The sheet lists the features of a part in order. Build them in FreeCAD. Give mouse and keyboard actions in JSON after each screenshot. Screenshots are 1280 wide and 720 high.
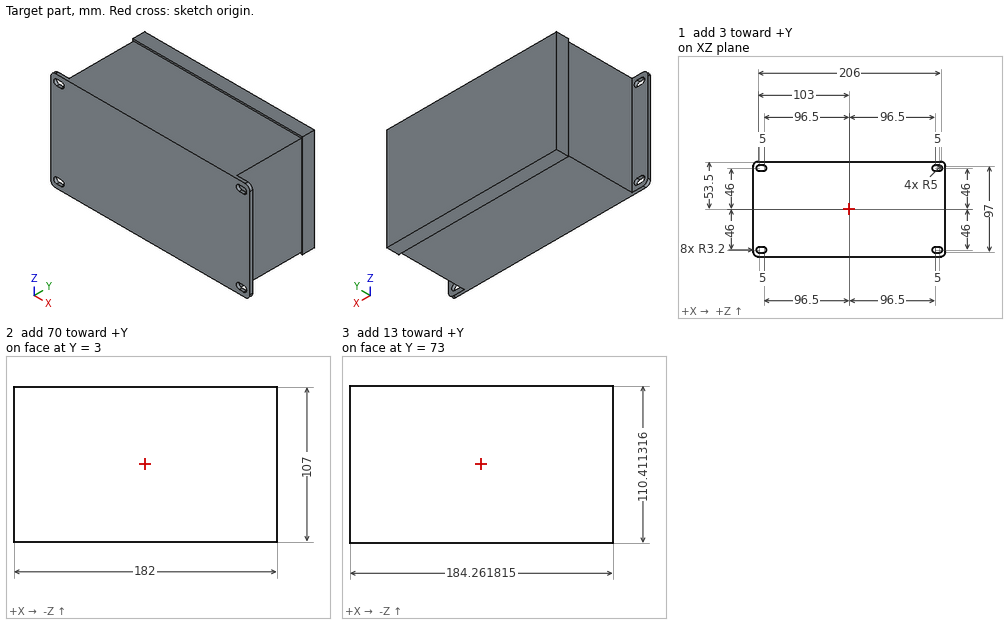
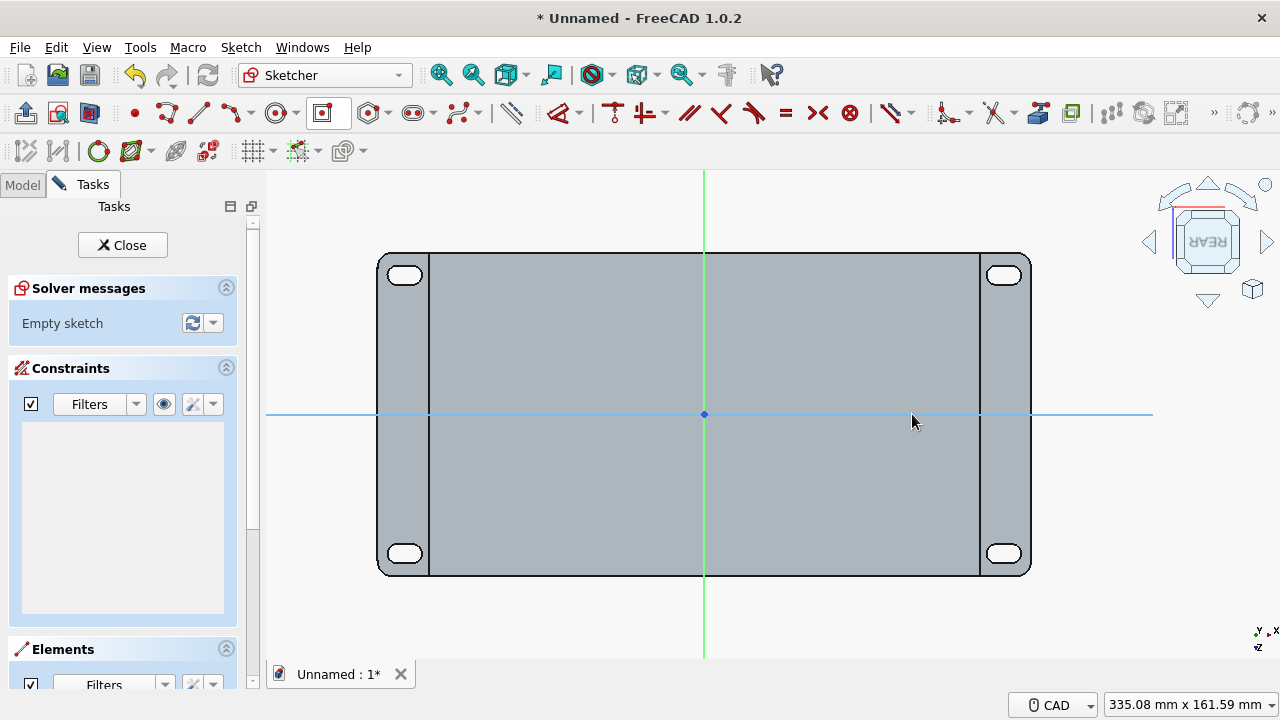
{"action": "left_click", "coordinate": [322, 114]}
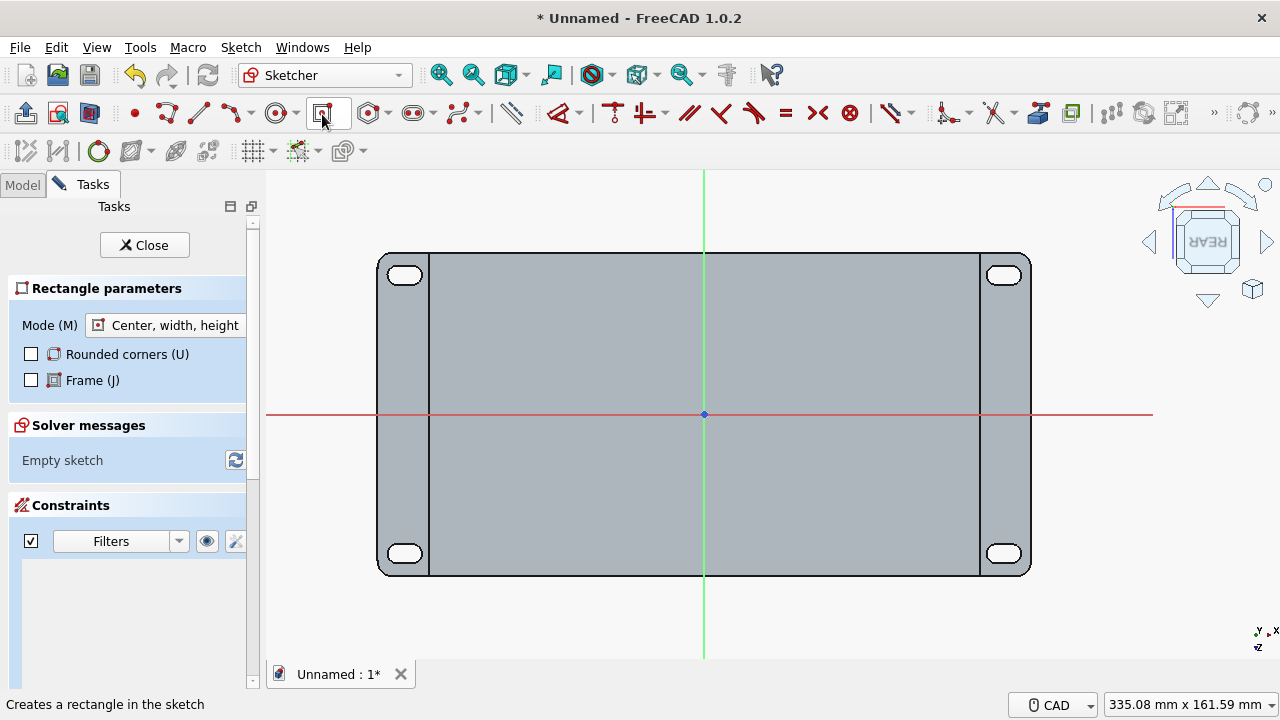
{"action": "left_click", "coordinate": [704, 414]}
{"action": "left_click", "coordinate": [983, 247]}
{"action": "key", "text": "Escape"}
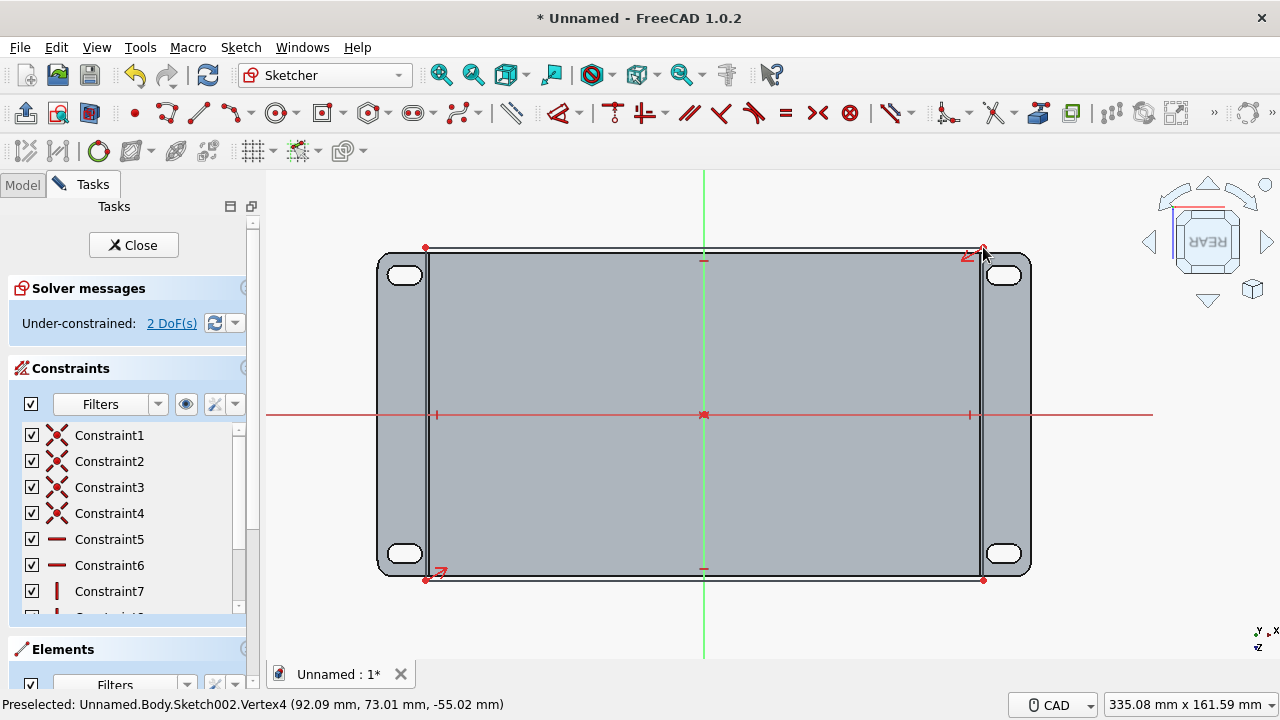
{"action": "left_click", "coordinate": [558, 114]}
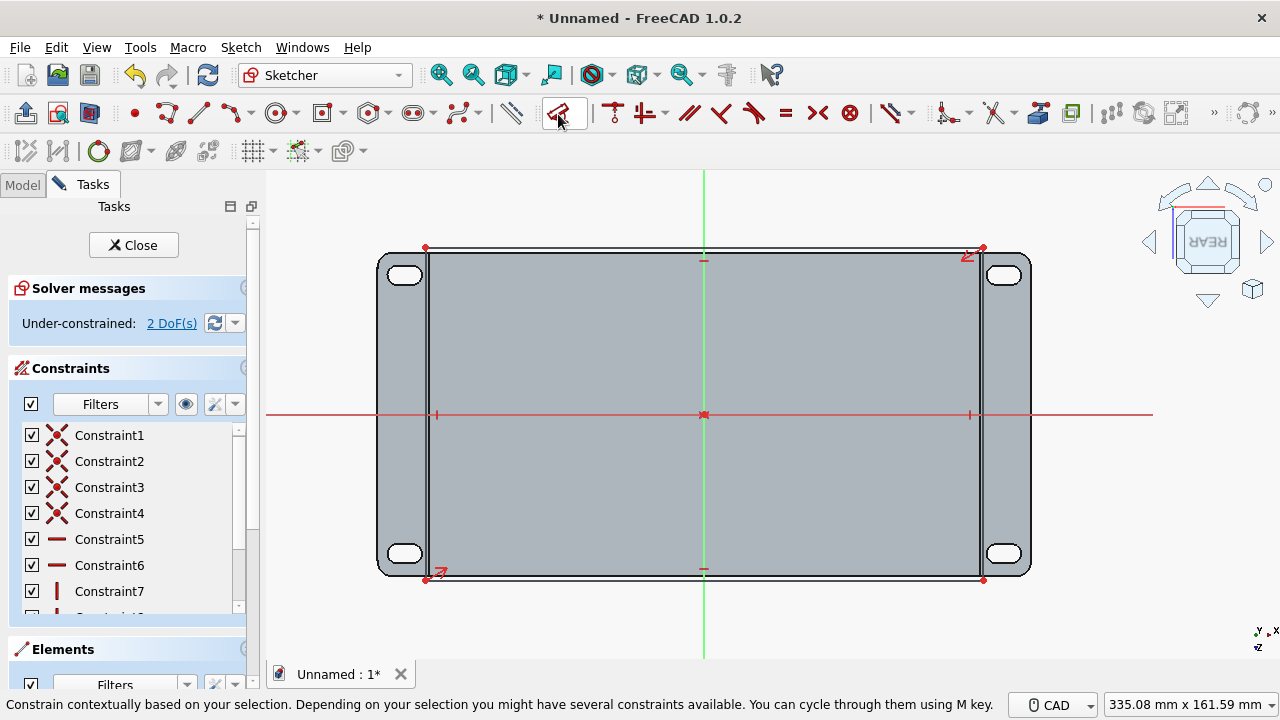
{"action": "left_click", "coordinate": [593, 581]}
{"action": "left_click", "coordinate": [576, 615]}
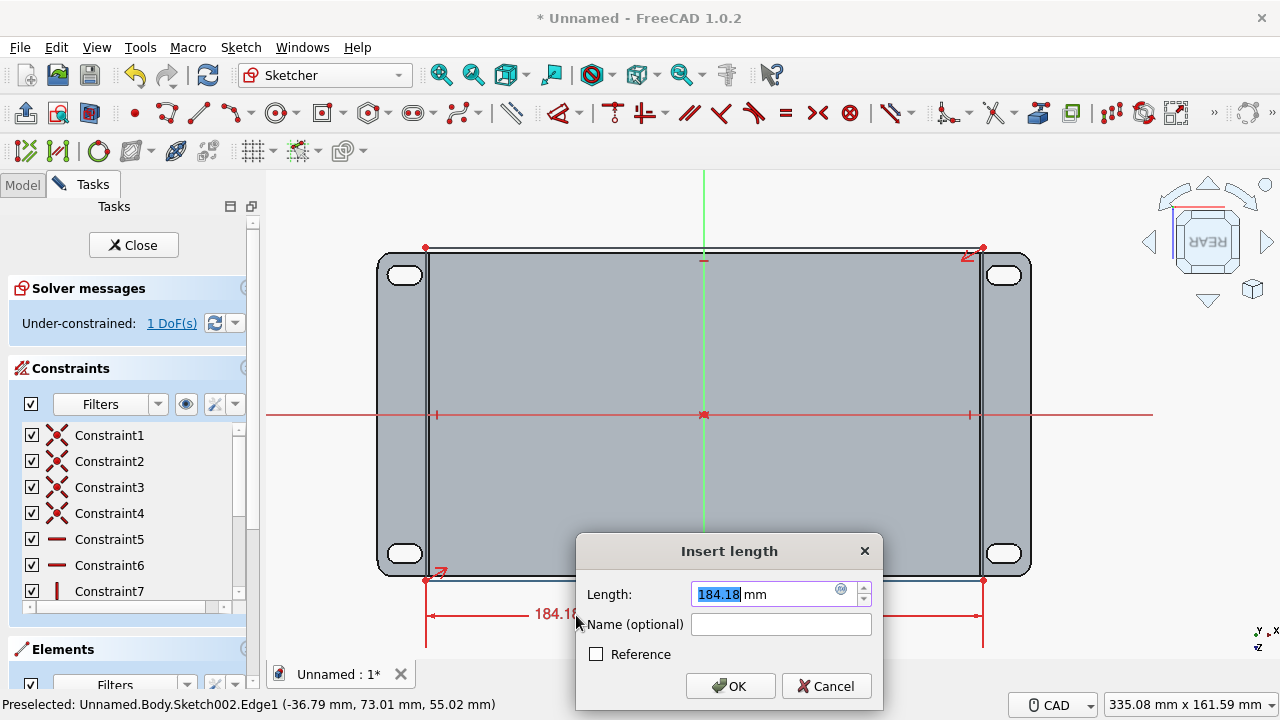
{"action": "type", "text": "184.261815"}
{"action": "key", "text": "Return"}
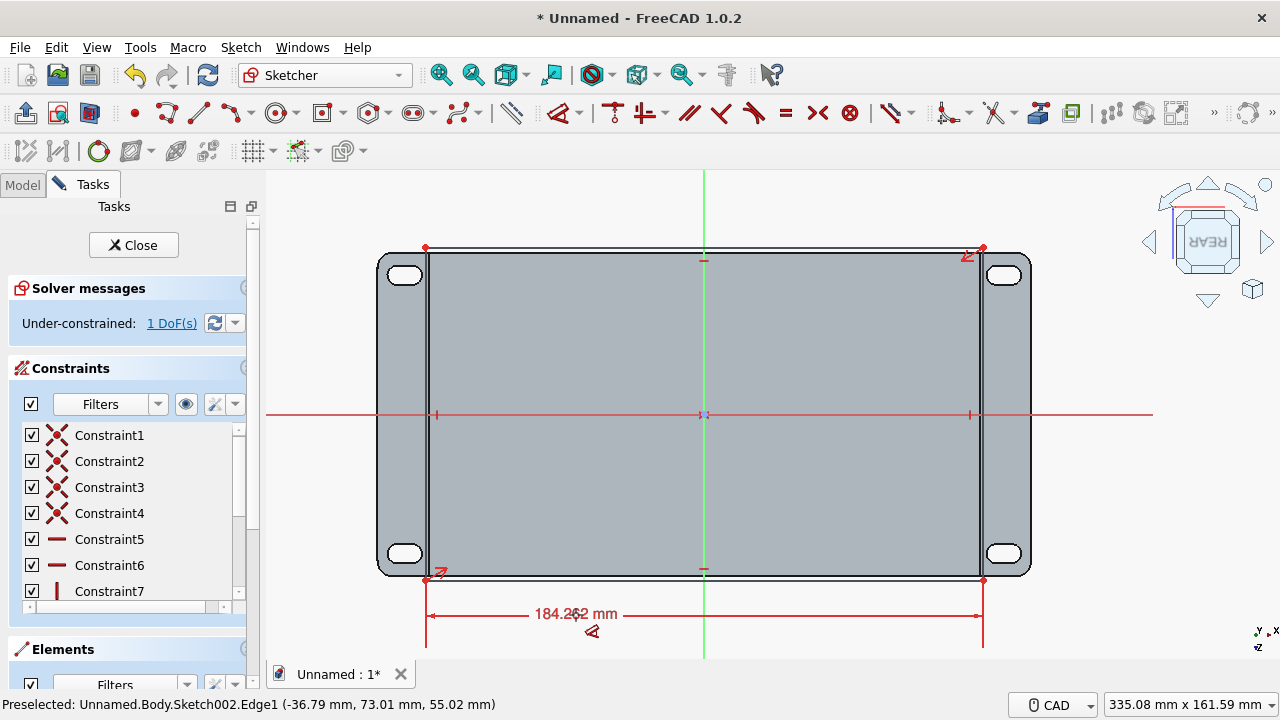
{"action": "left_click", "coordinate": [983, 481]}
{"action": "left_click", "coordinate": [1017, 338]}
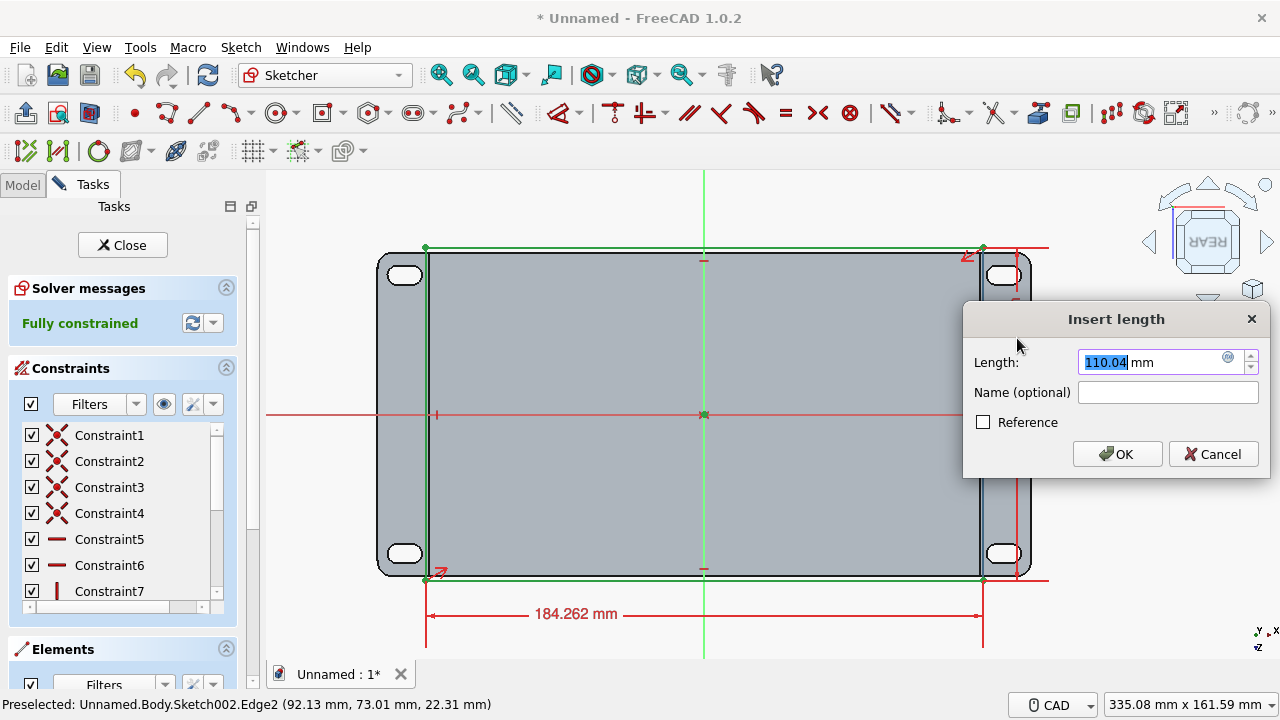
{"action": "type", "text": "110.411316"}
{"action": "key", "text": "Return"}
{"action": "key", "text": "Escape"}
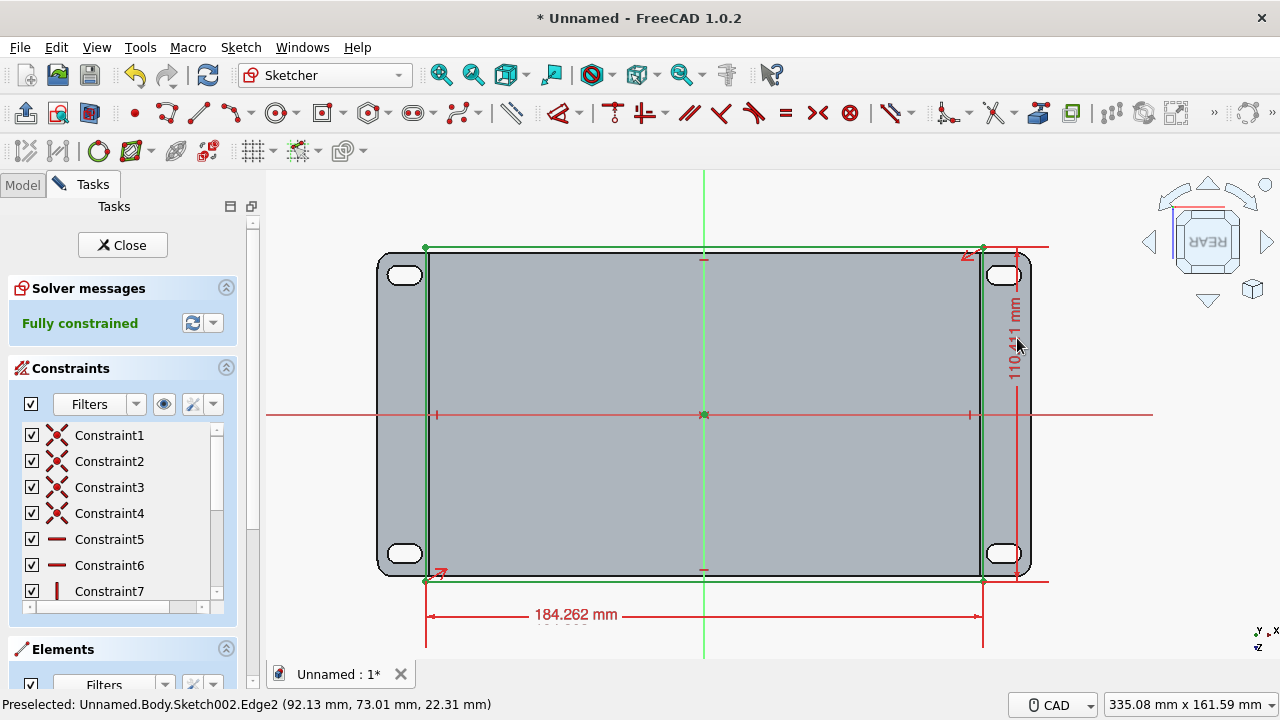
{"action": "left_click", "coordinate": [123, 245]}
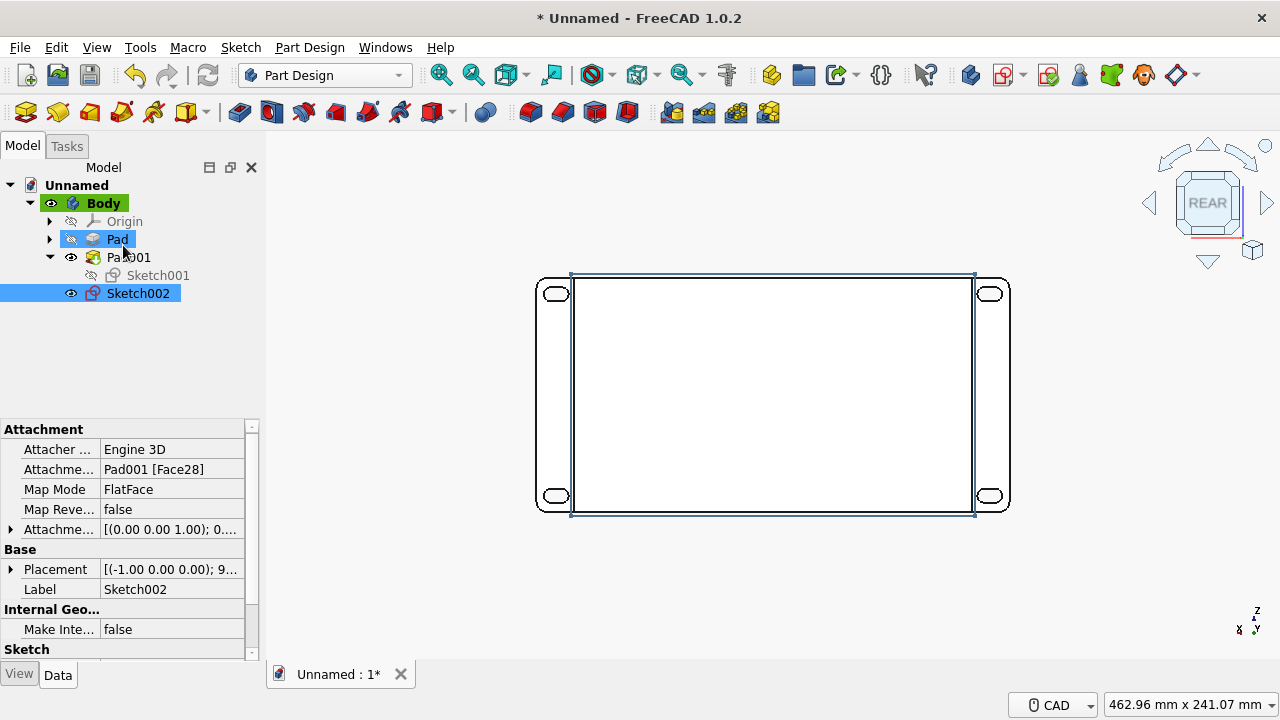
{"action": "left_click", "coordinate": [26, 112]}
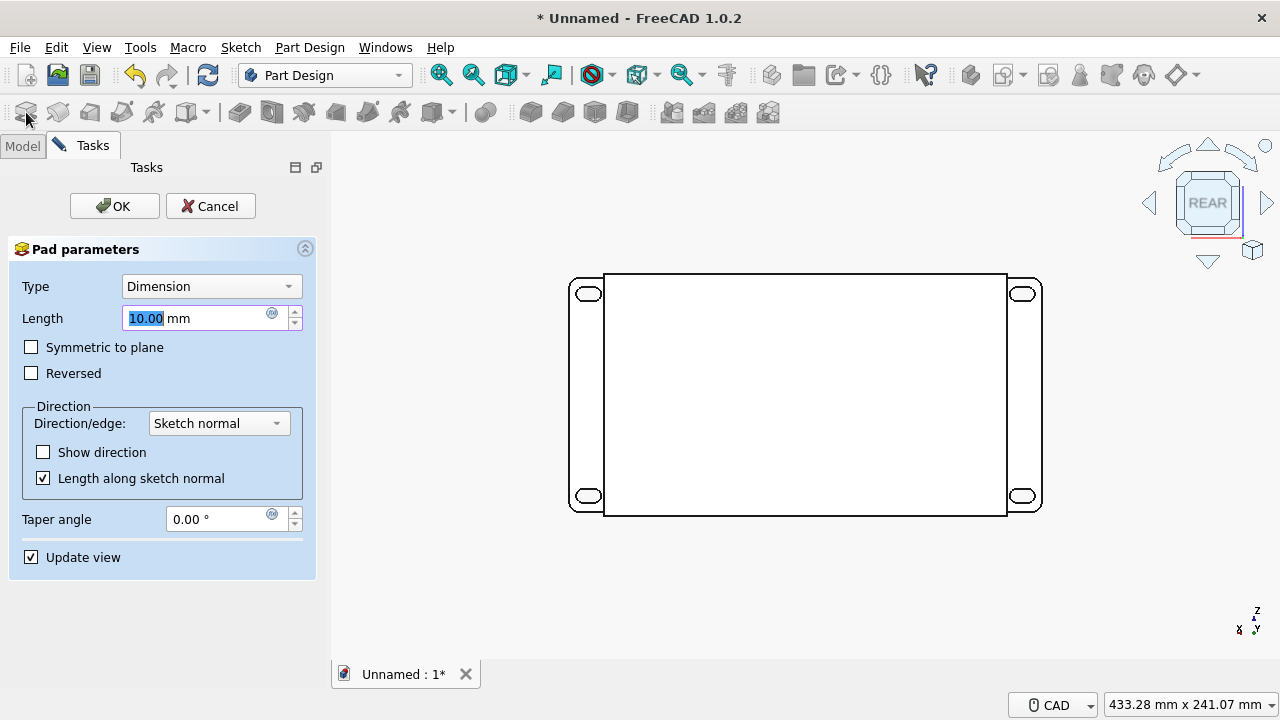
{"action": "type", "text": "13"}
{"action": "key", "text": "Tab"}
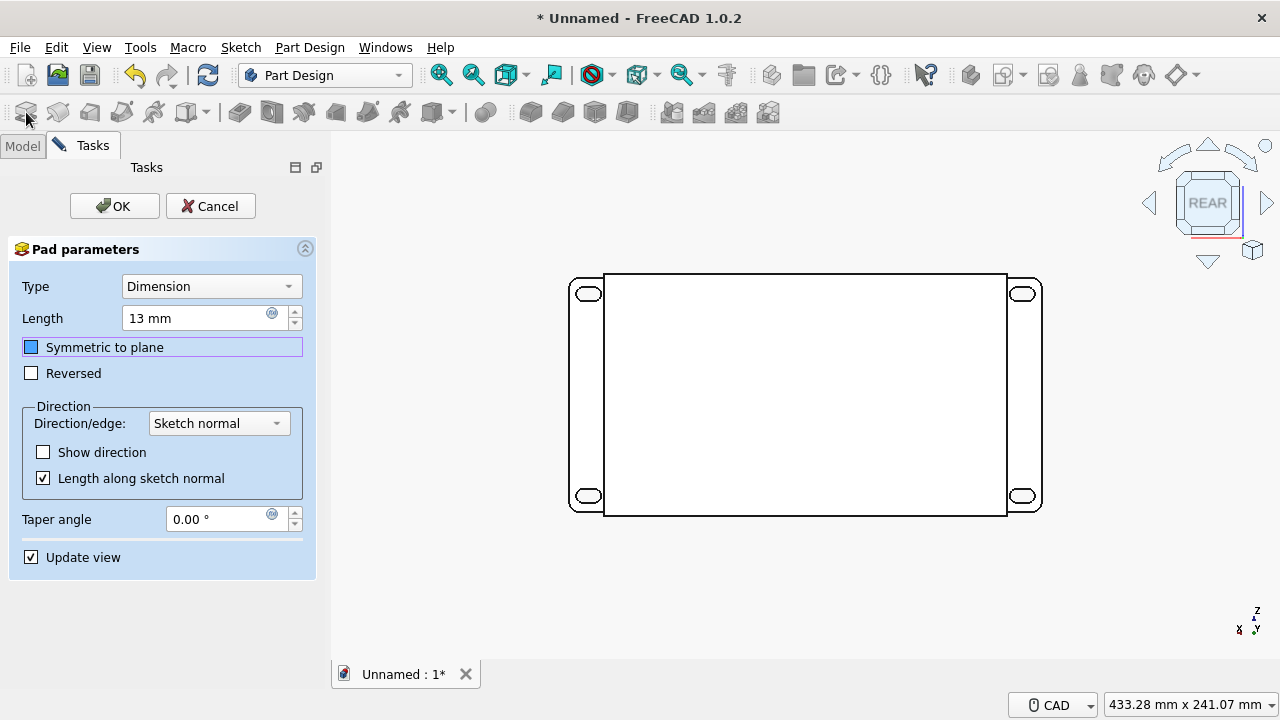
{"action": "left_click", "coordinate": [115, 206]}